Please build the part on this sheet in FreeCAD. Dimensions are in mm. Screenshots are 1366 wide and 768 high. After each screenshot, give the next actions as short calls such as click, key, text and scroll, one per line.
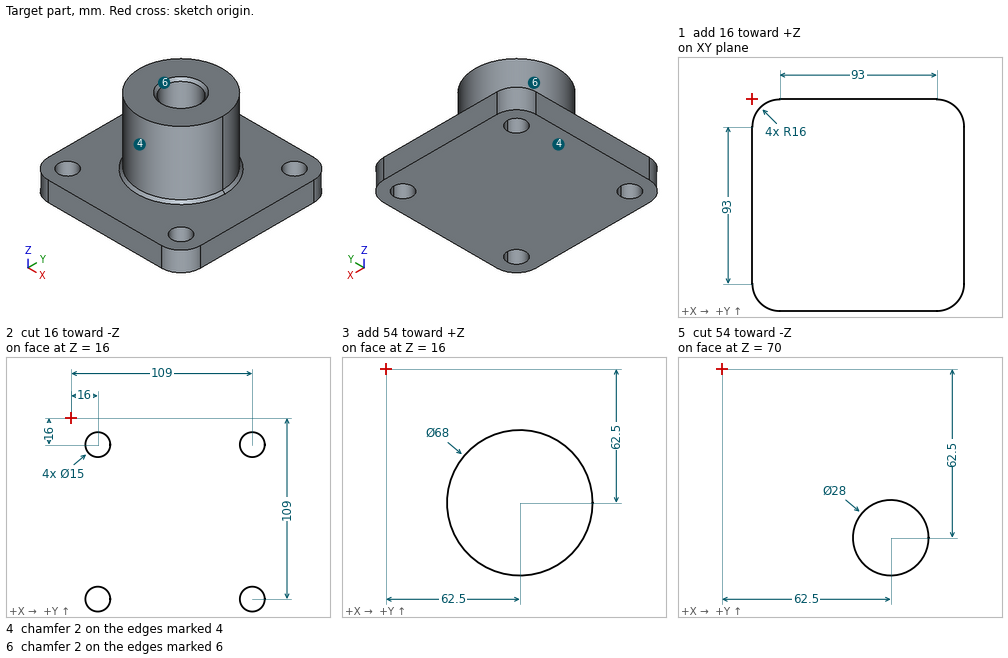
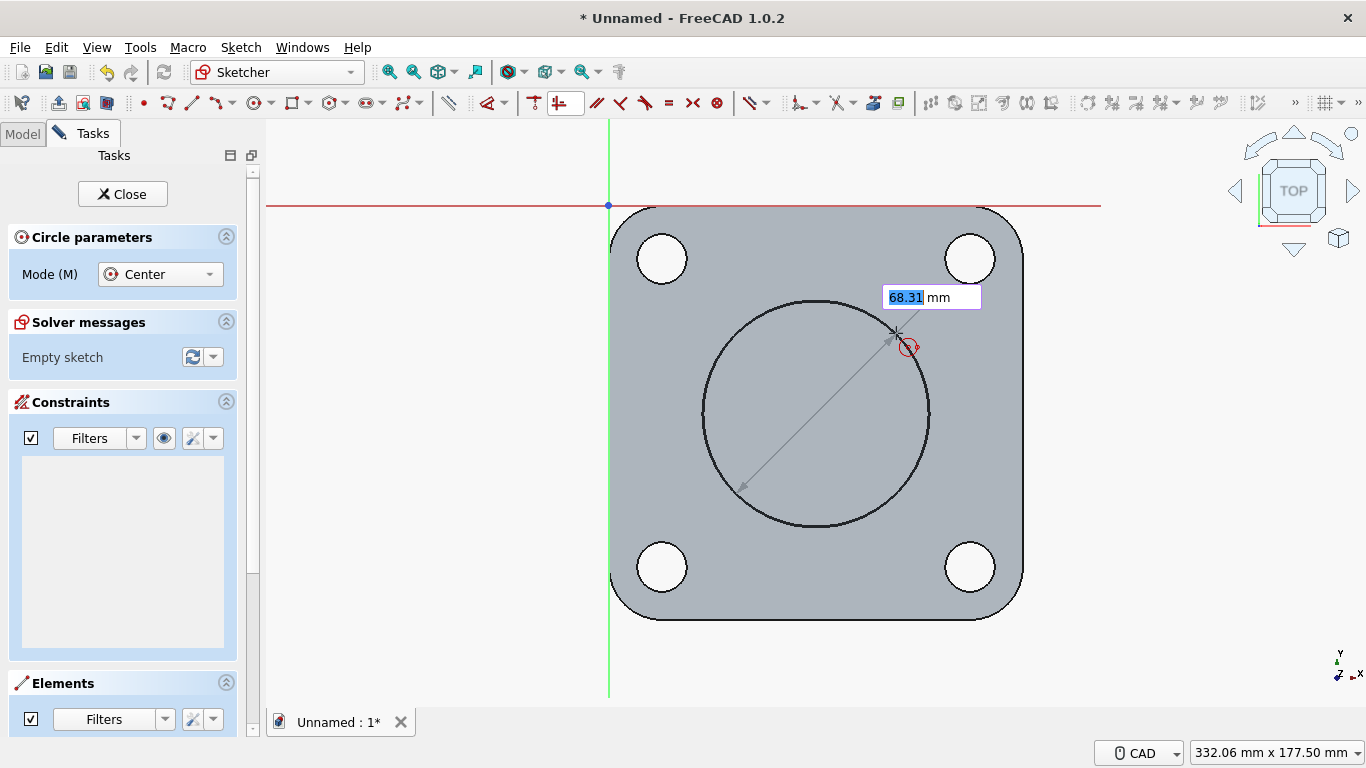
text(68)
key(Return)
key(Escape)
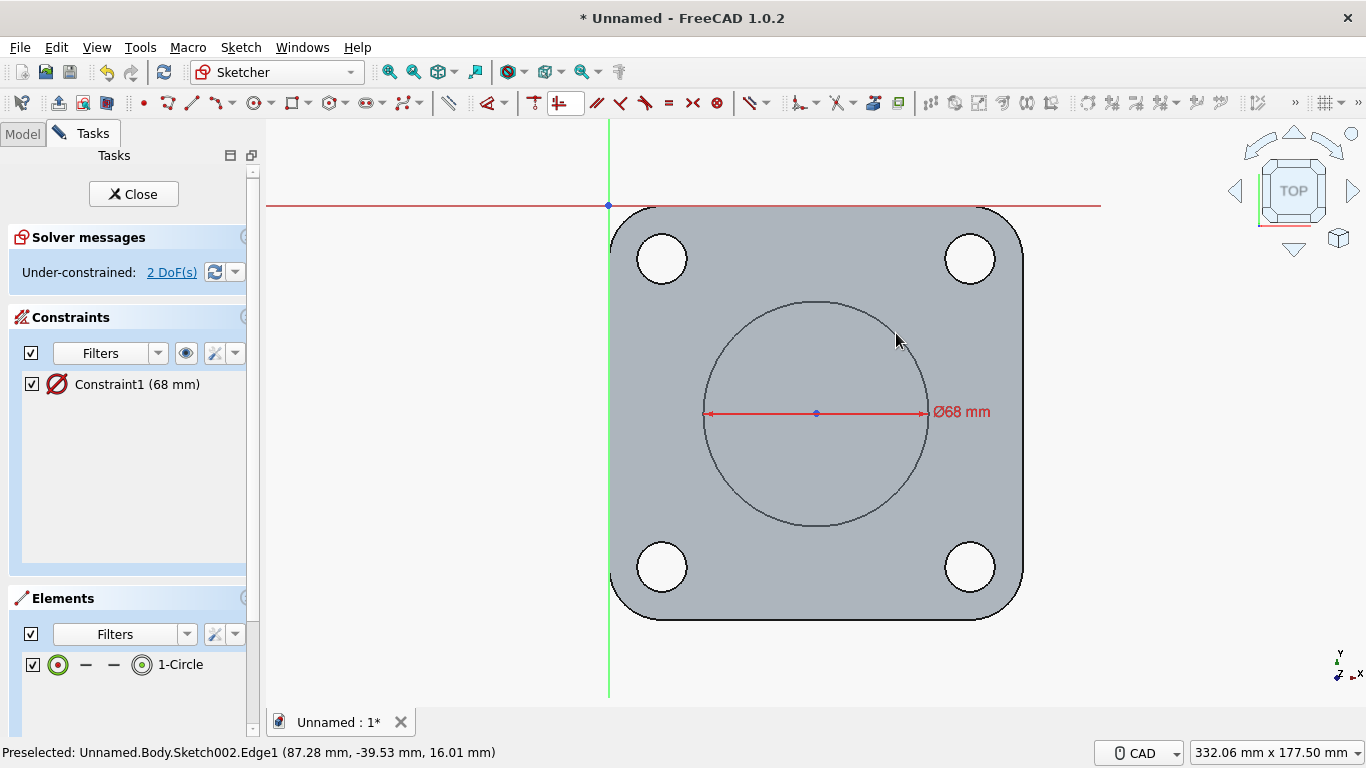
key(d)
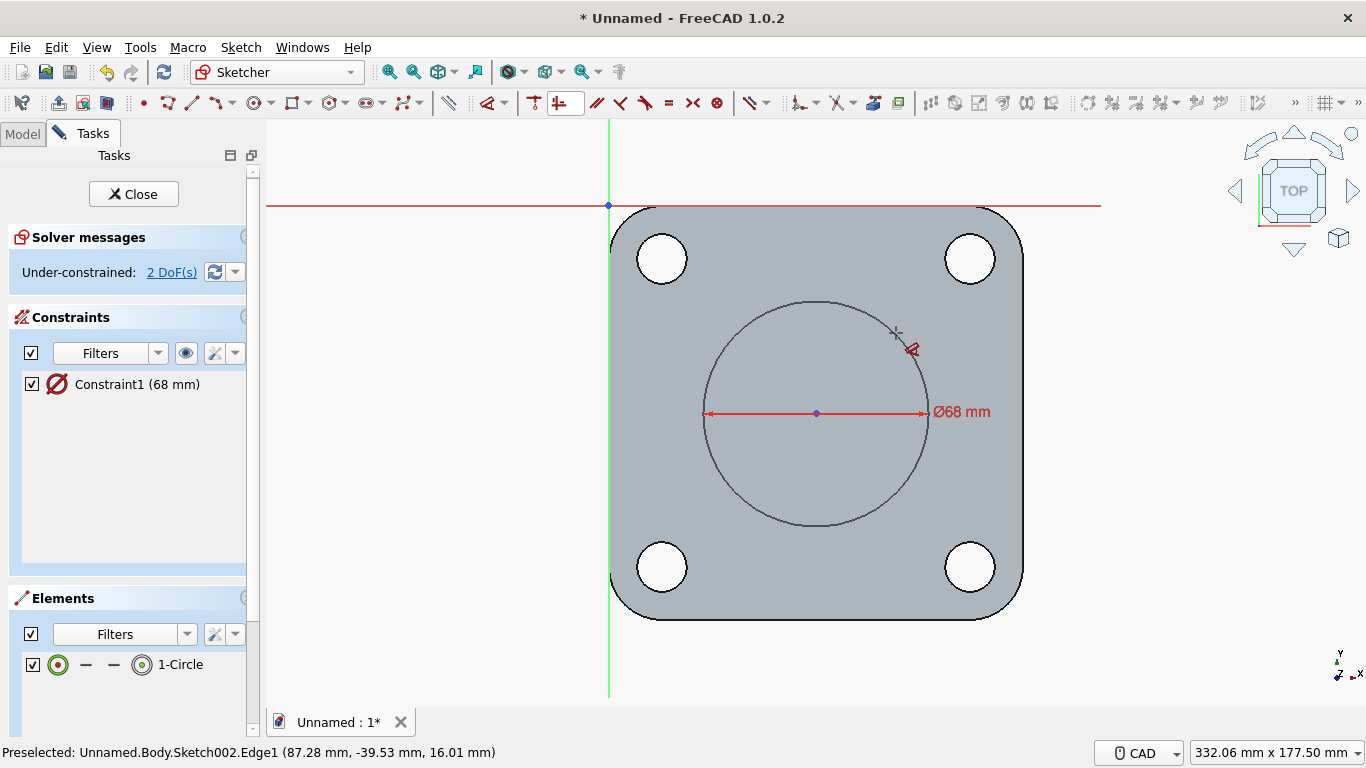
click(816, 414)
click(712, 172)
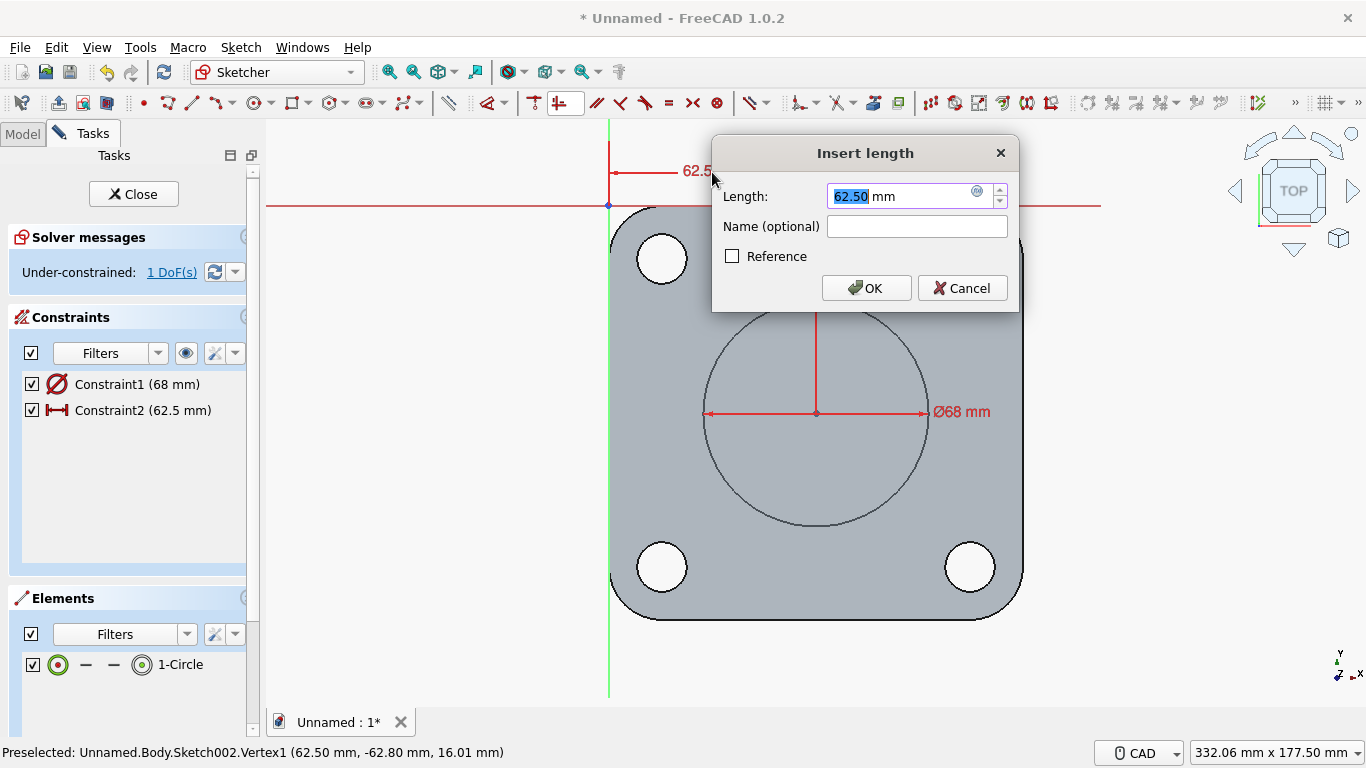
text(62.5)
key(Return)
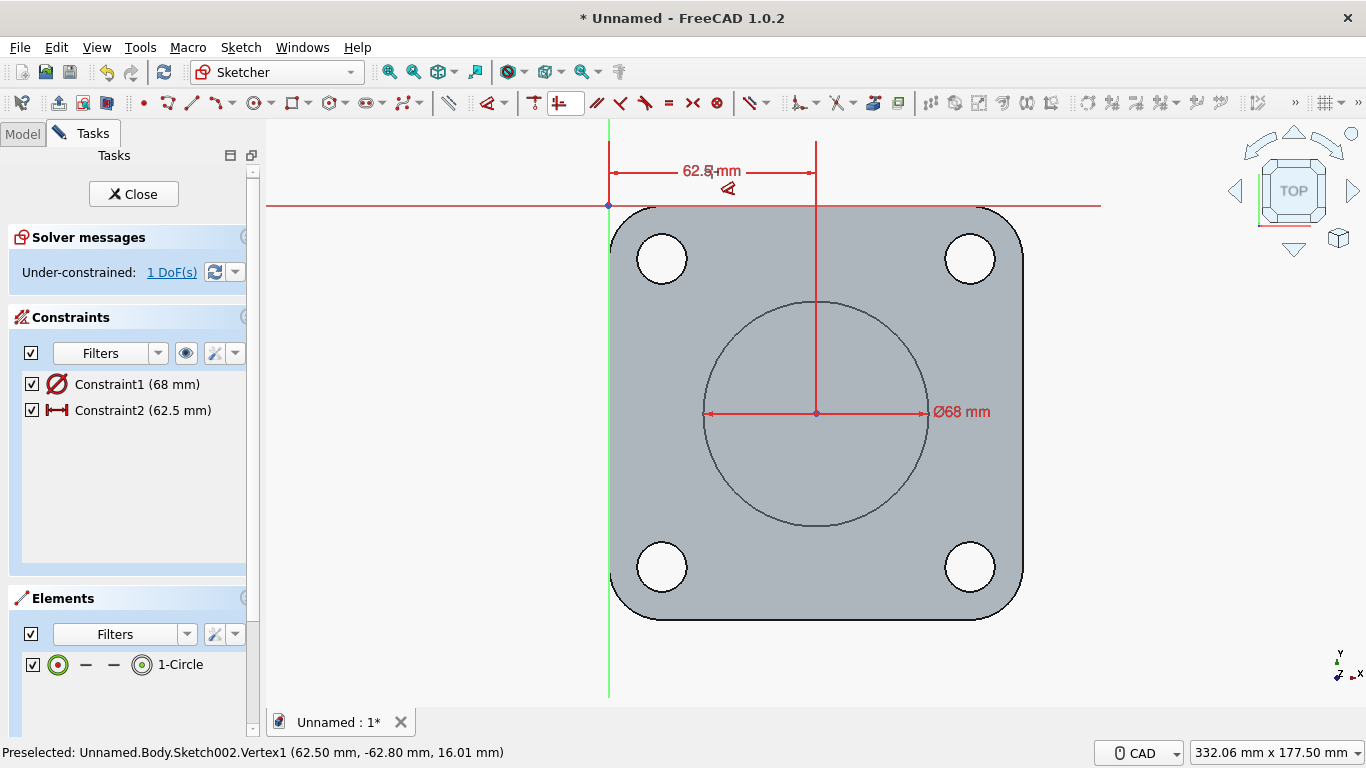
click(816, 414)
click(575, 310)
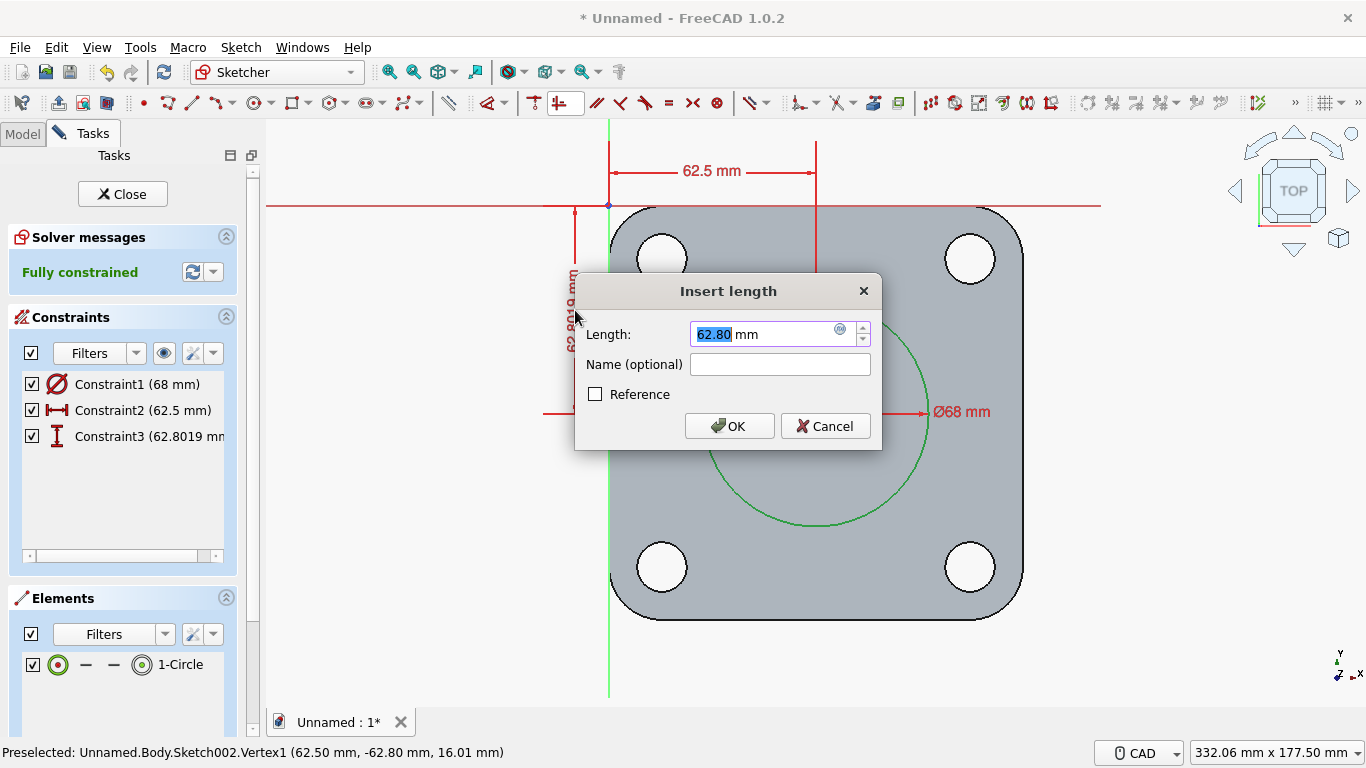
text(62.5)
key(Return)
key(Escape)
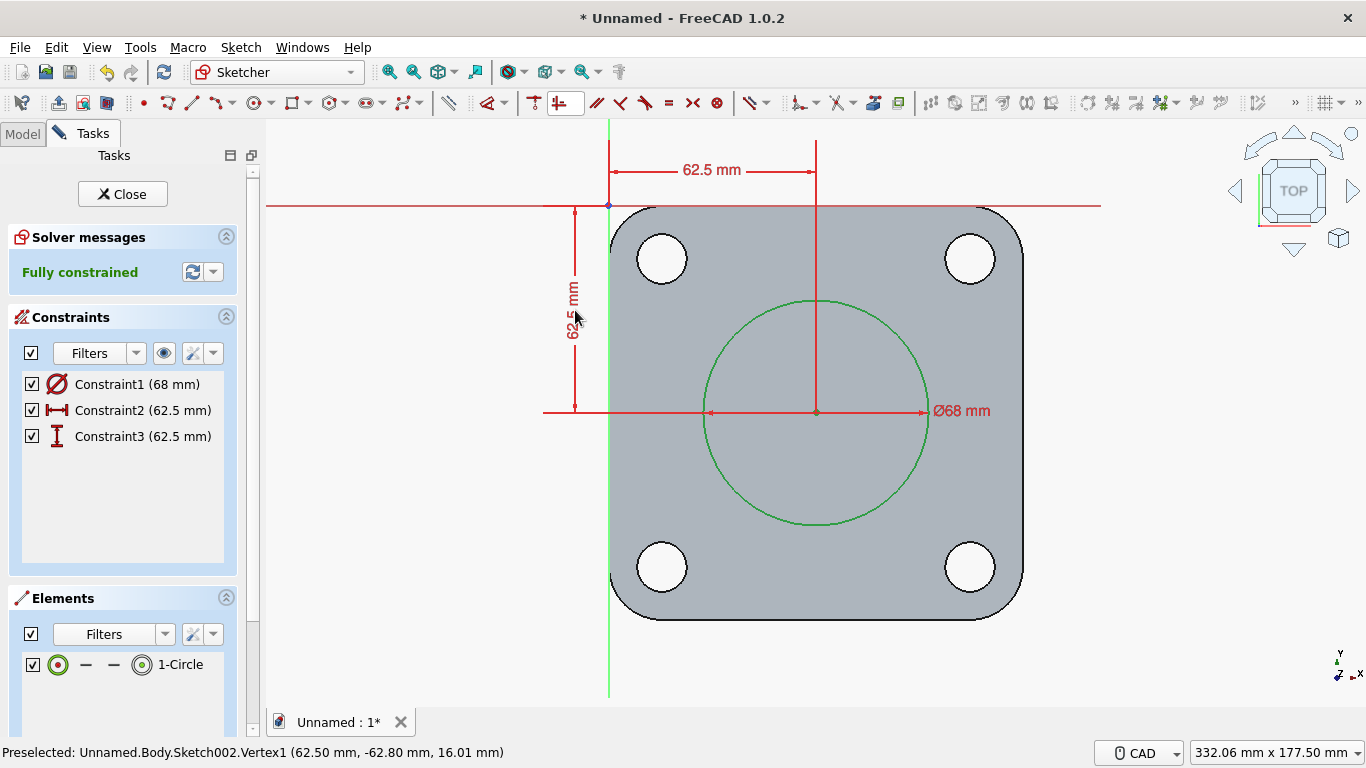
click(123, 194)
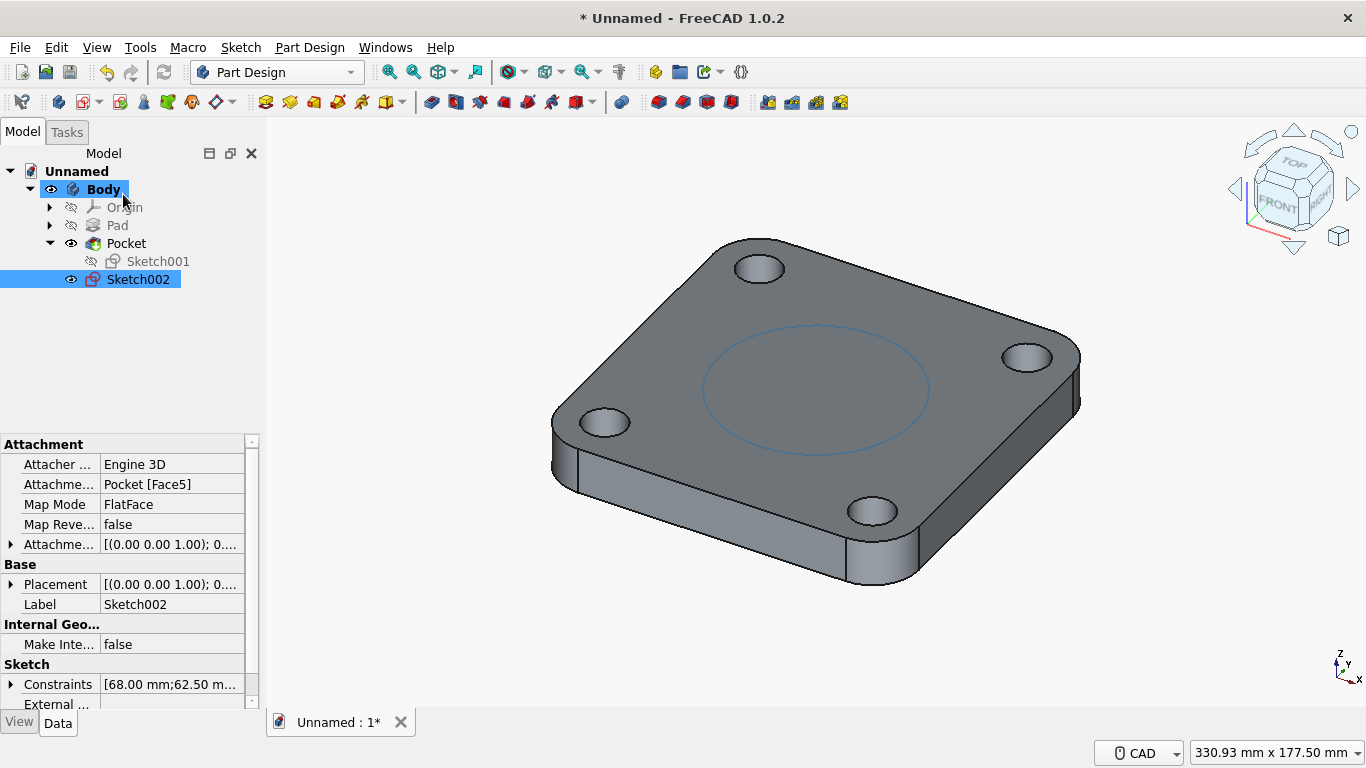
click(266, 102)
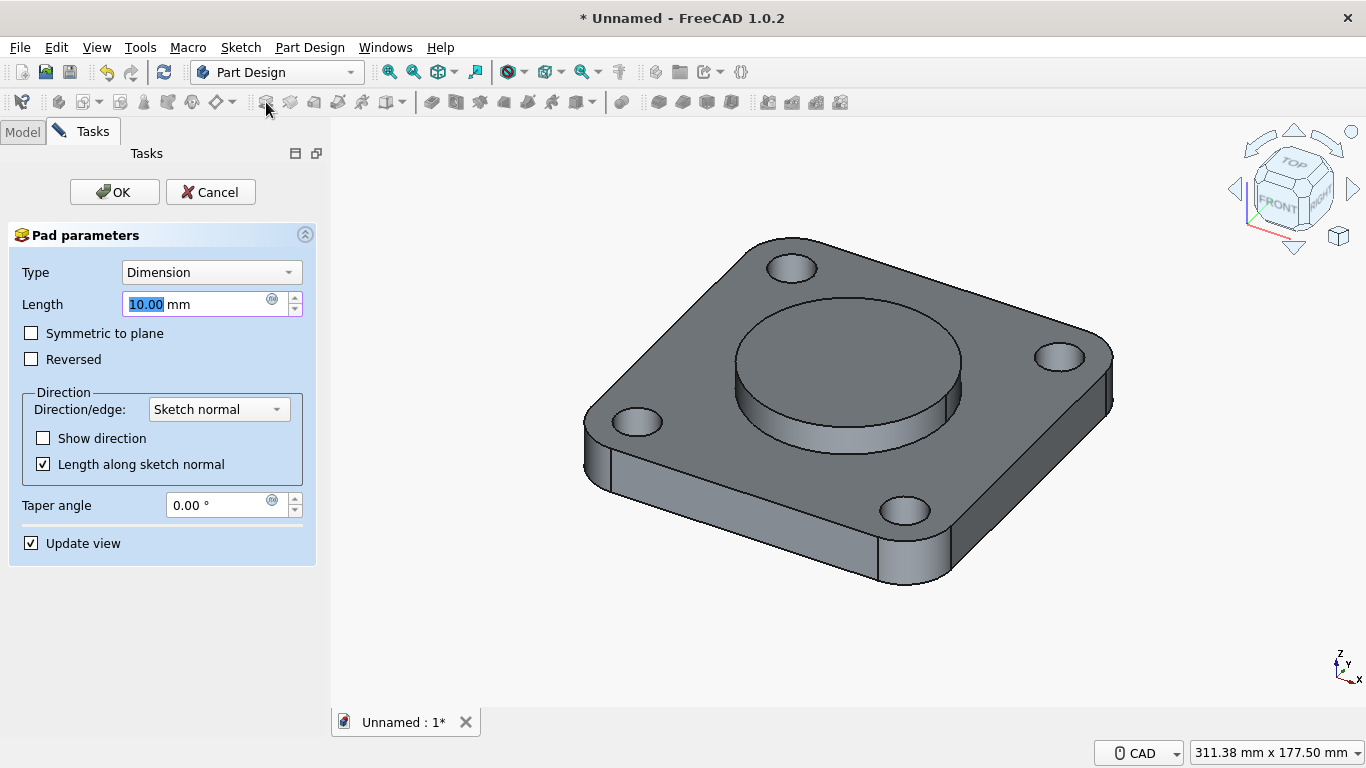
text(54)
key(Tab)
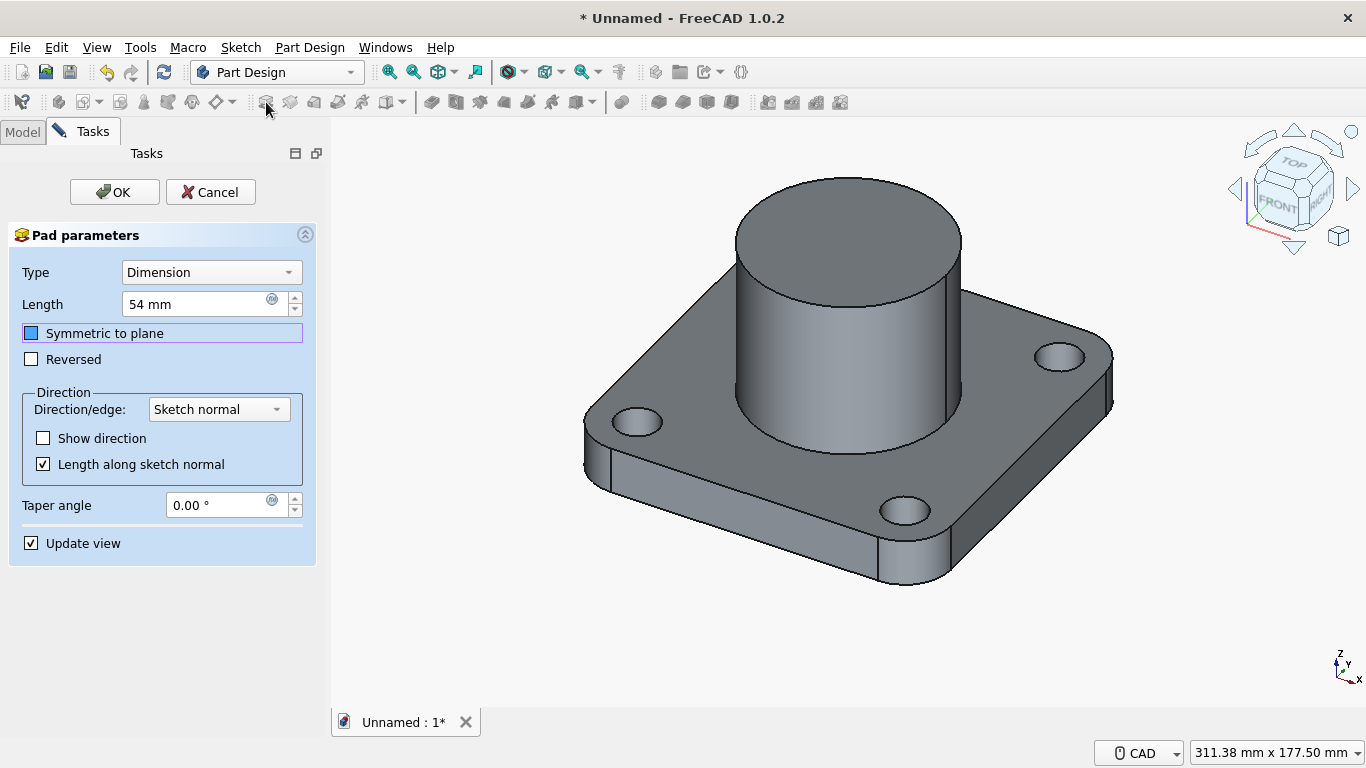
click(115, 192)